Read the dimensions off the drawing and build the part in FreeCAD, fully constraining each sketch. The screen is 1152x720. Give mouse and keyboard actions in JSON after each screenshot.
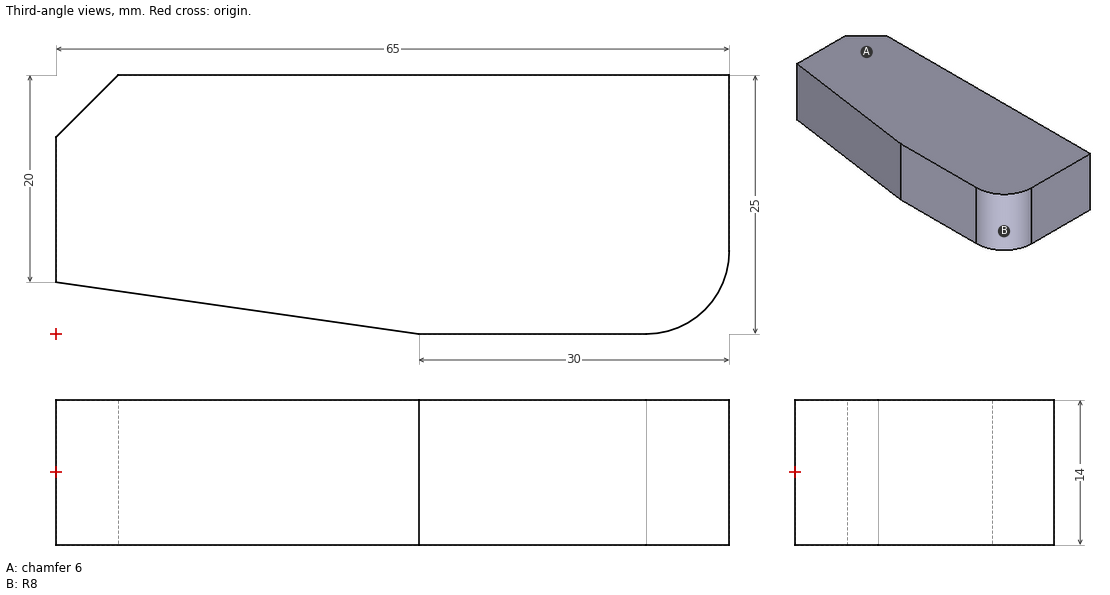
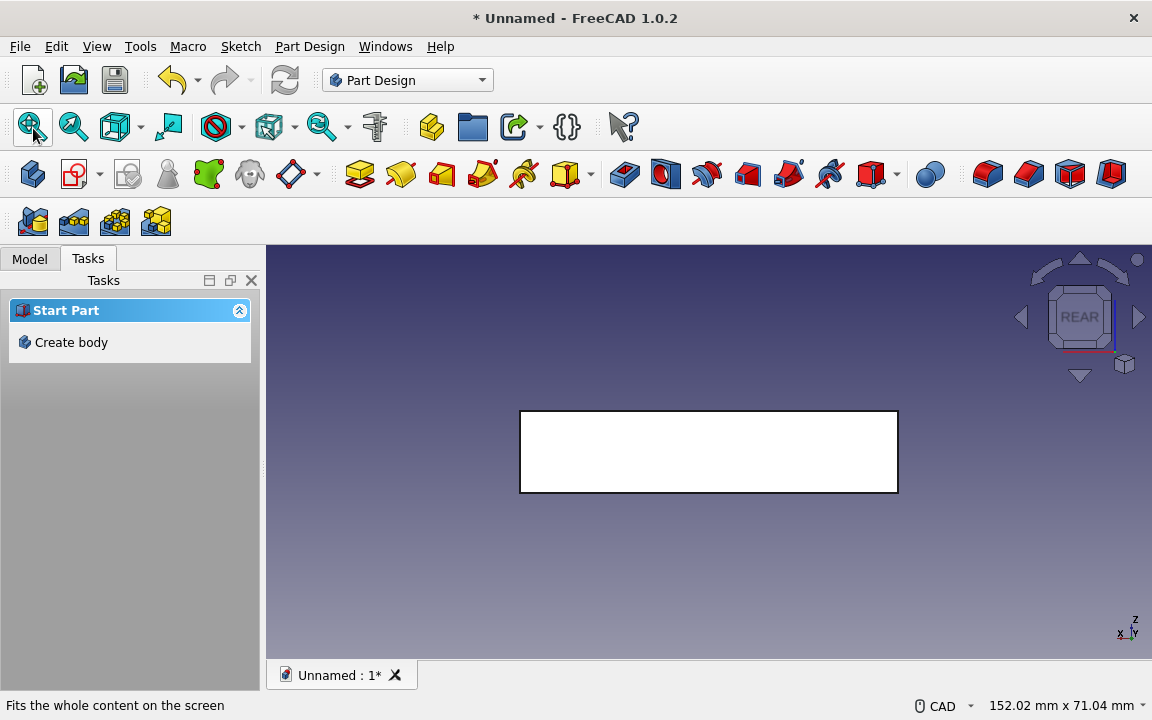
{"action": "left_click", "coordinate": [898, 451]}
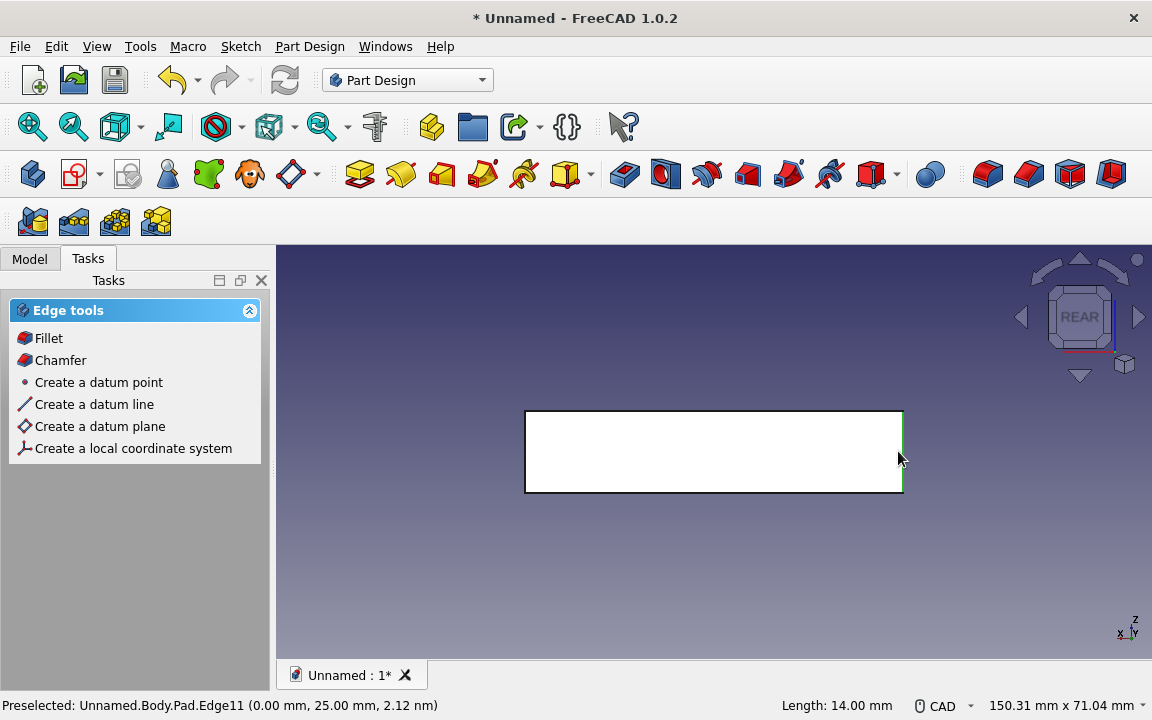
{"action": "left_click", "coordinate": [1029, 174]}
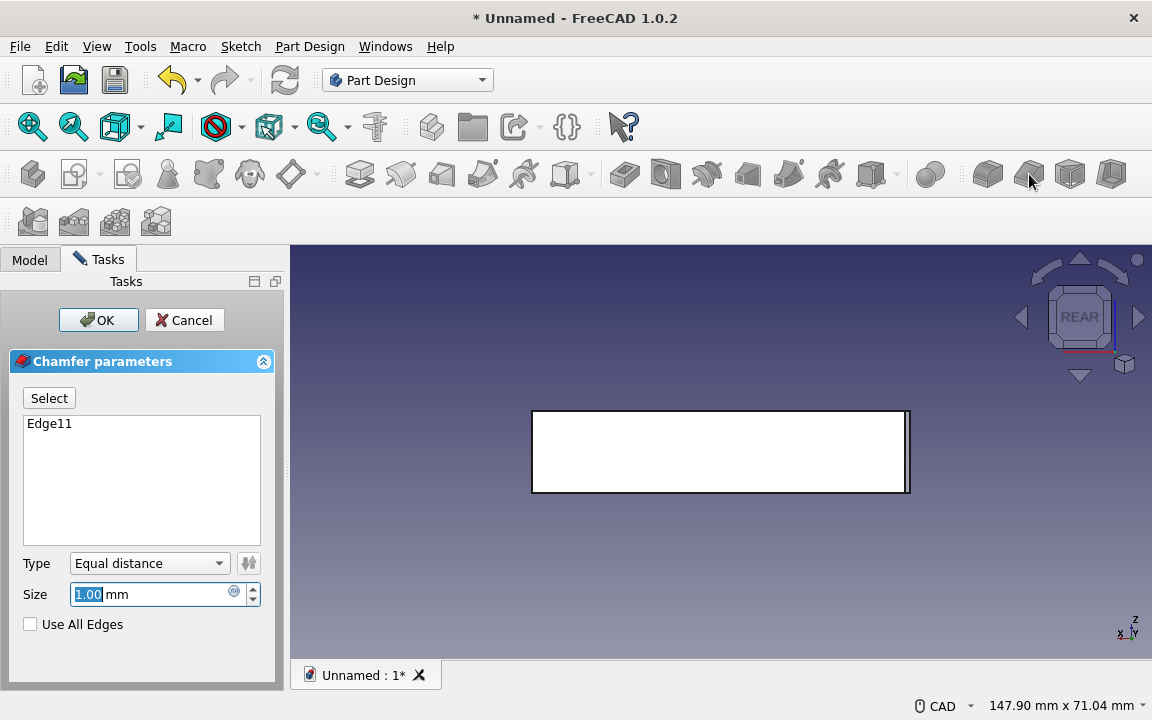
{"action": "type", "text": "6"}
{"action": "key", "text": "Tab"}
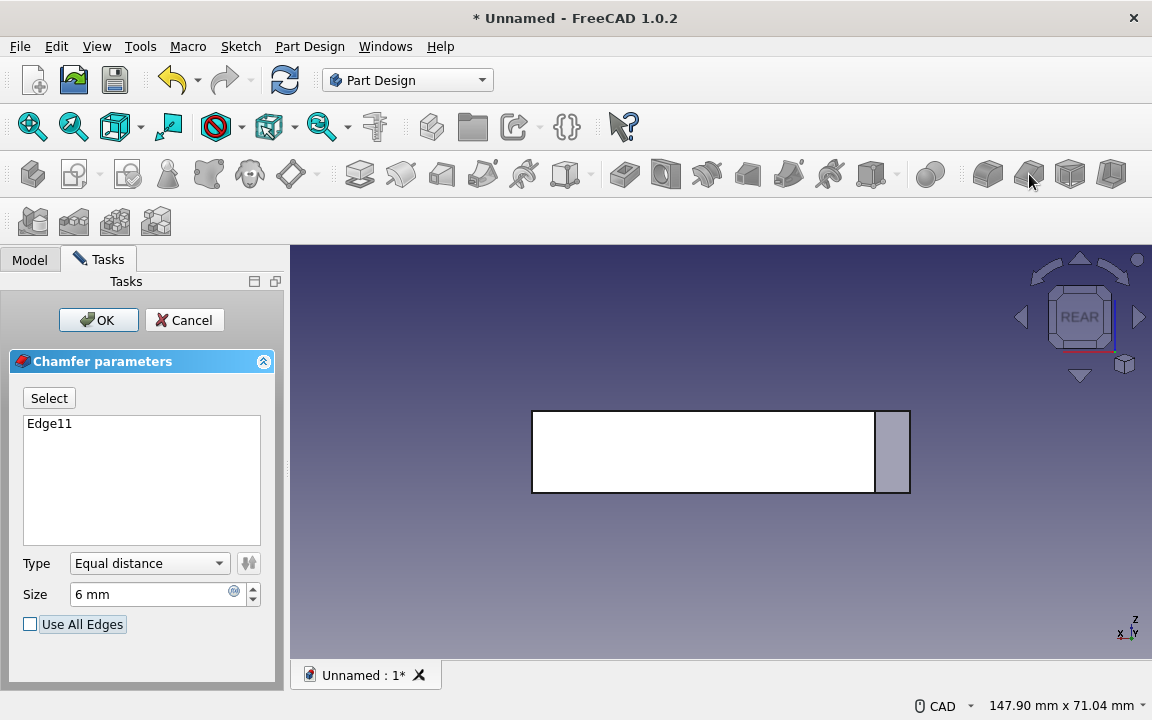
{"action": "left_click", "coordinate": [99, 320]}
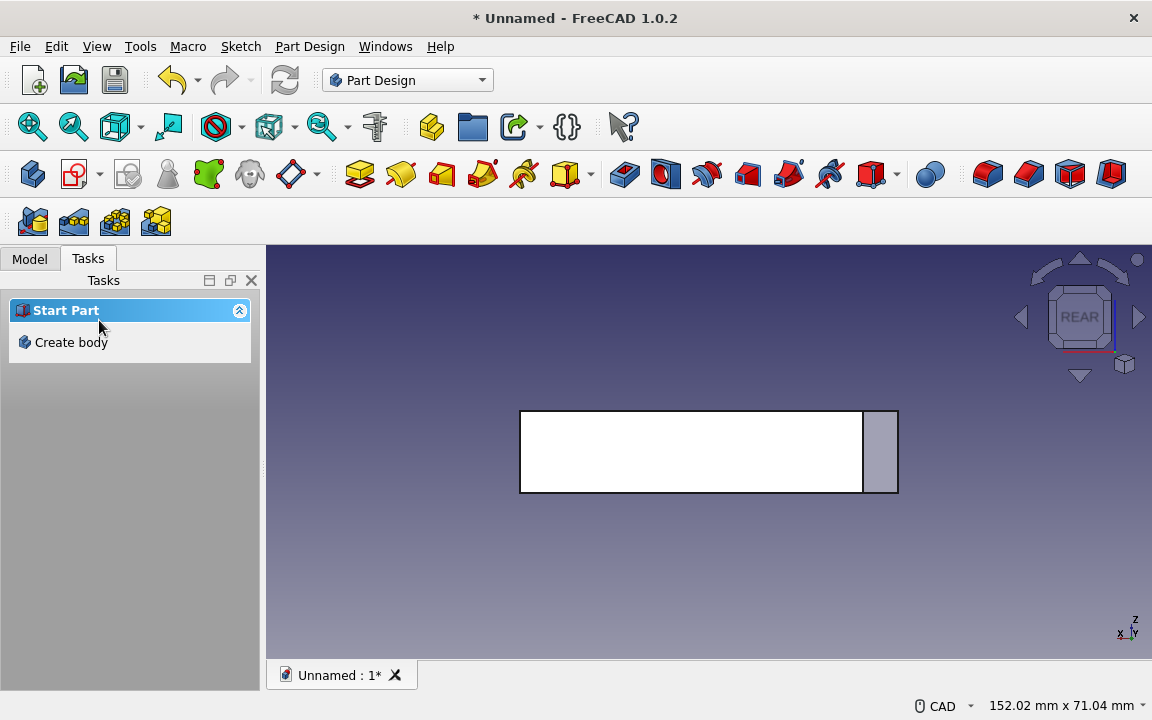
{"action": "left_click", "coordinate": [33, 128]}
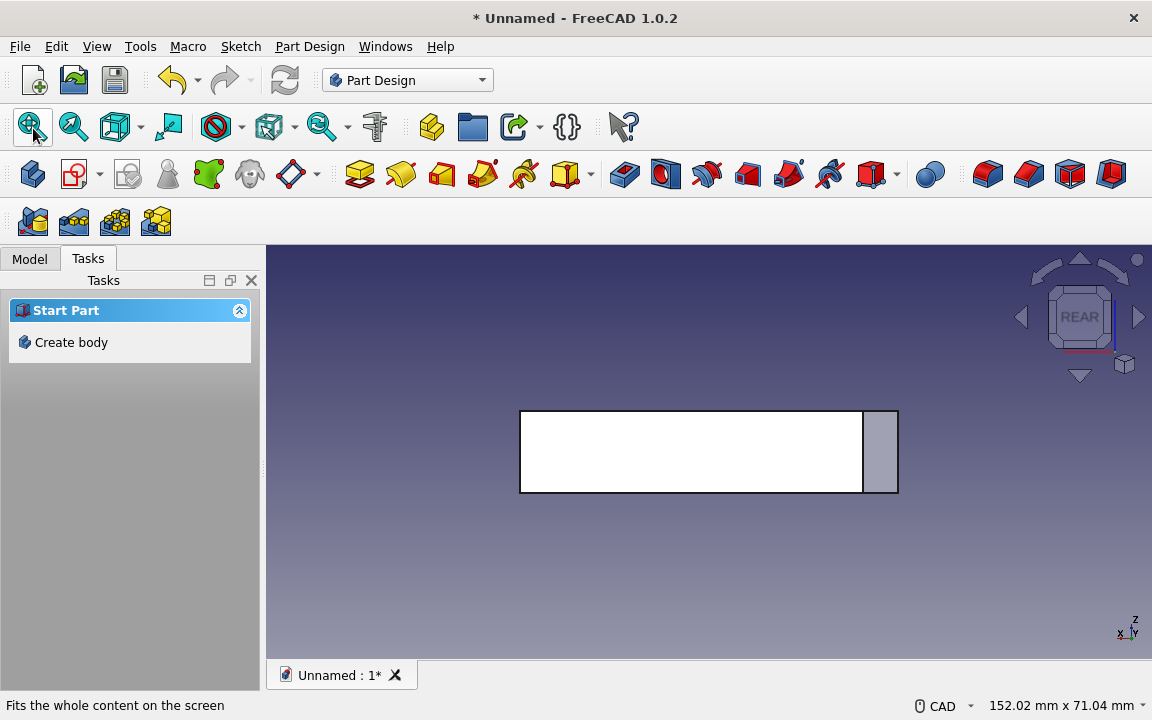
{"action": "key", "text": "0"}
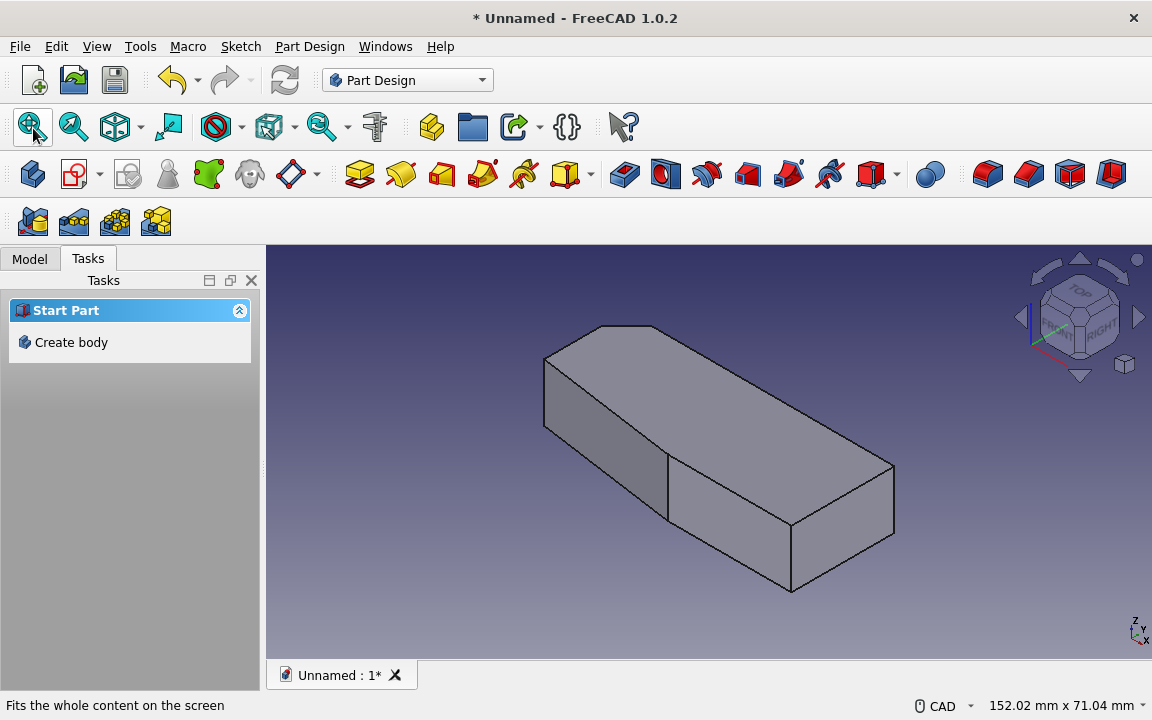
{"action": "left_click", "coordinate": [791, 558]}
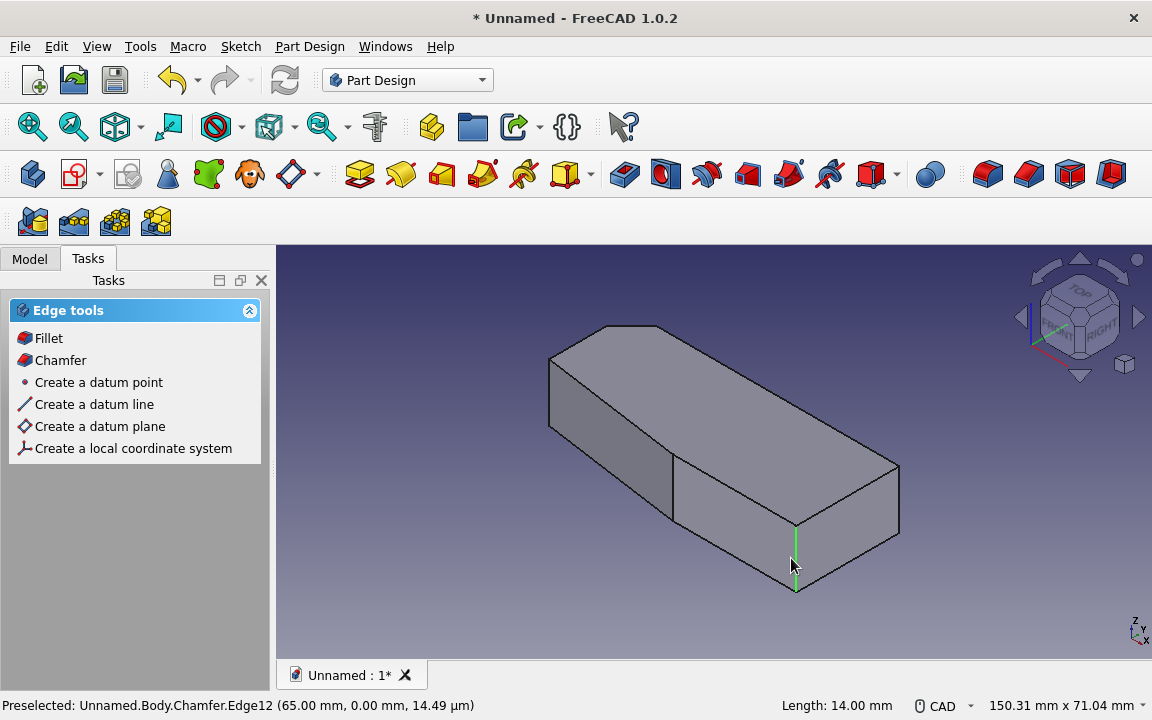
{"action": "left_click", "coordinate": [988, 174]}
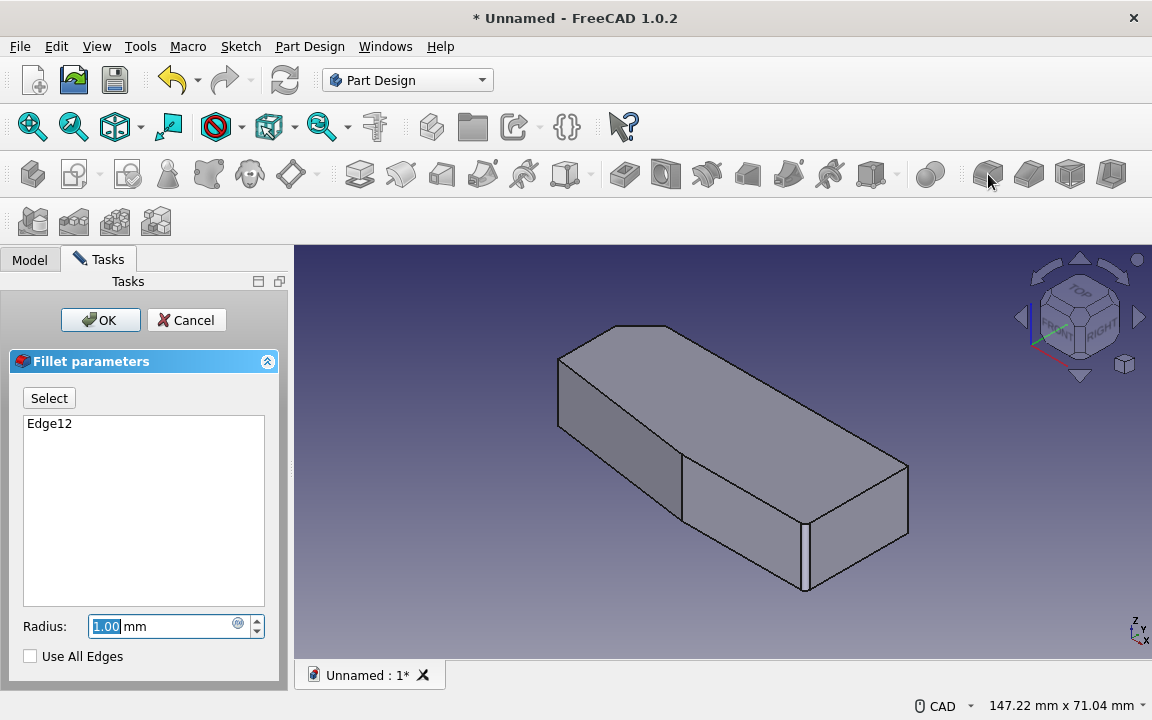
{"action": "type", "text": "8"}
{"action": "key", "text": "Tab"}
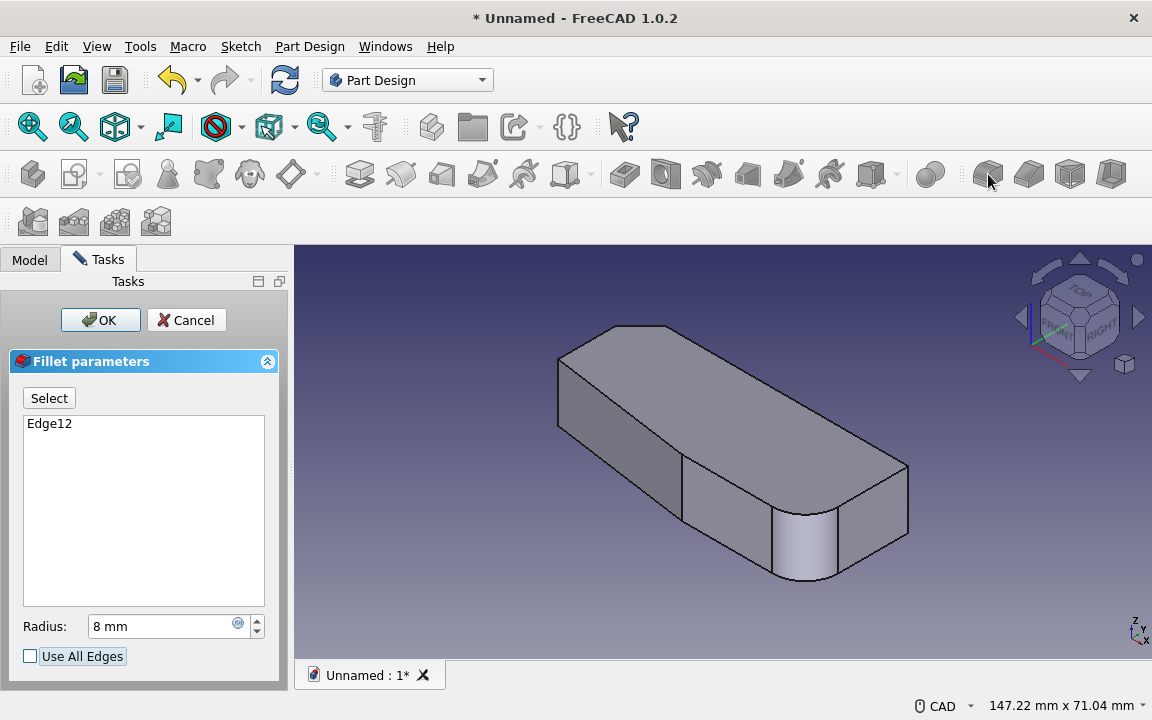
{"action": "left_click", "coordinate": [101, 320]}